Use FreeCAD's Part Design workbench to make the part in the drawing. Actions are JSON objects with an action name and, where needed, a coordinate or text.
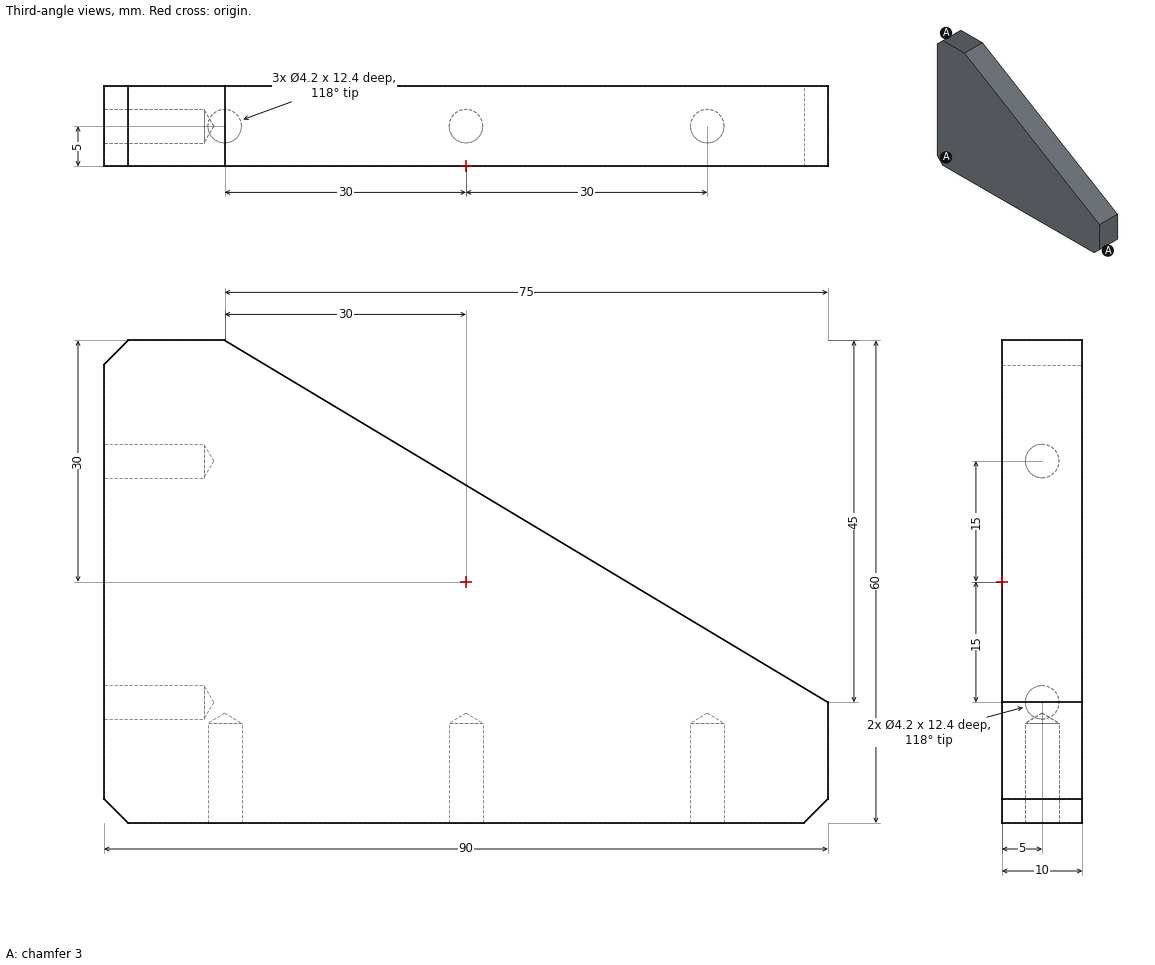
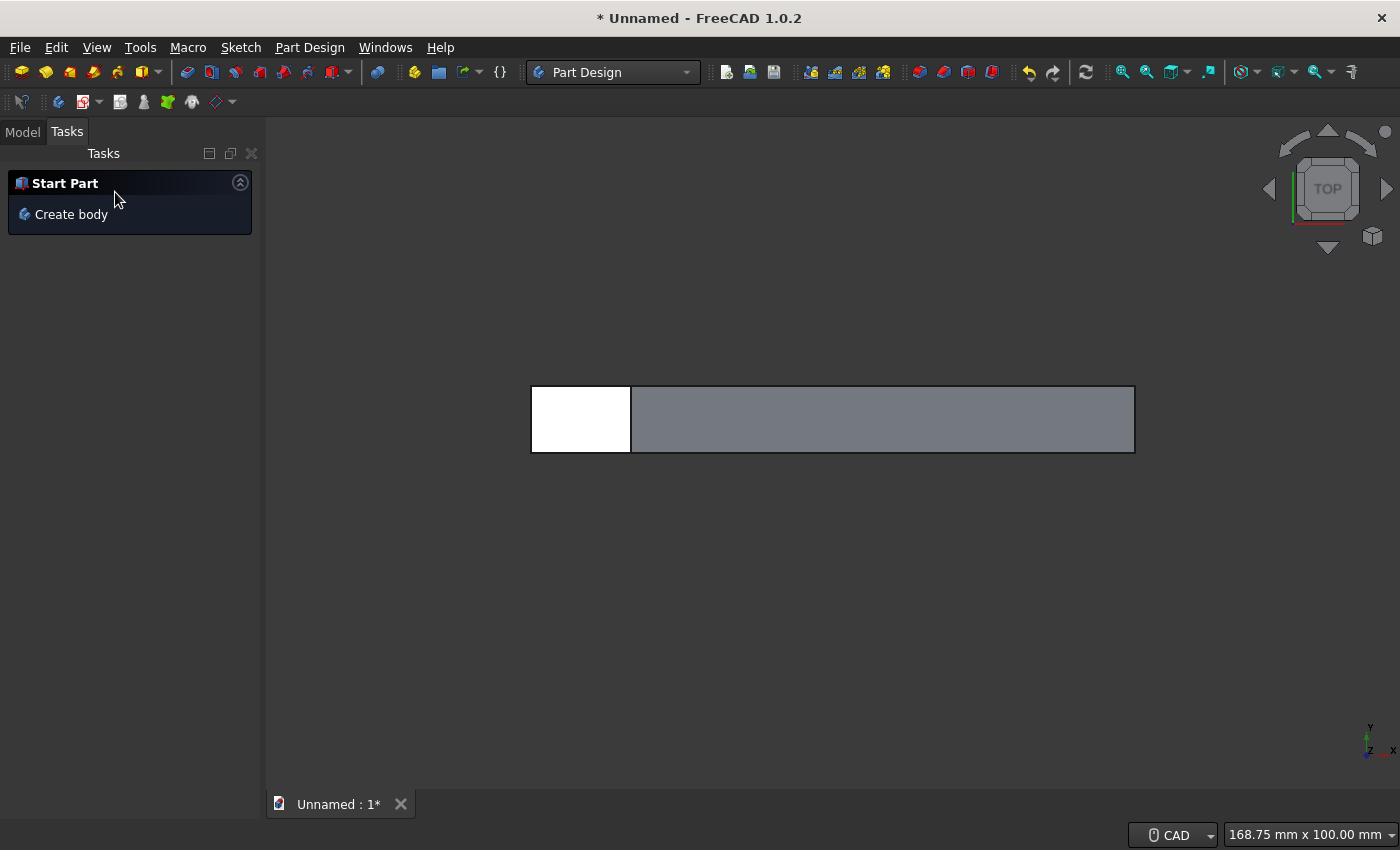
{"action": "left_click", "coordinate": [531, 418]}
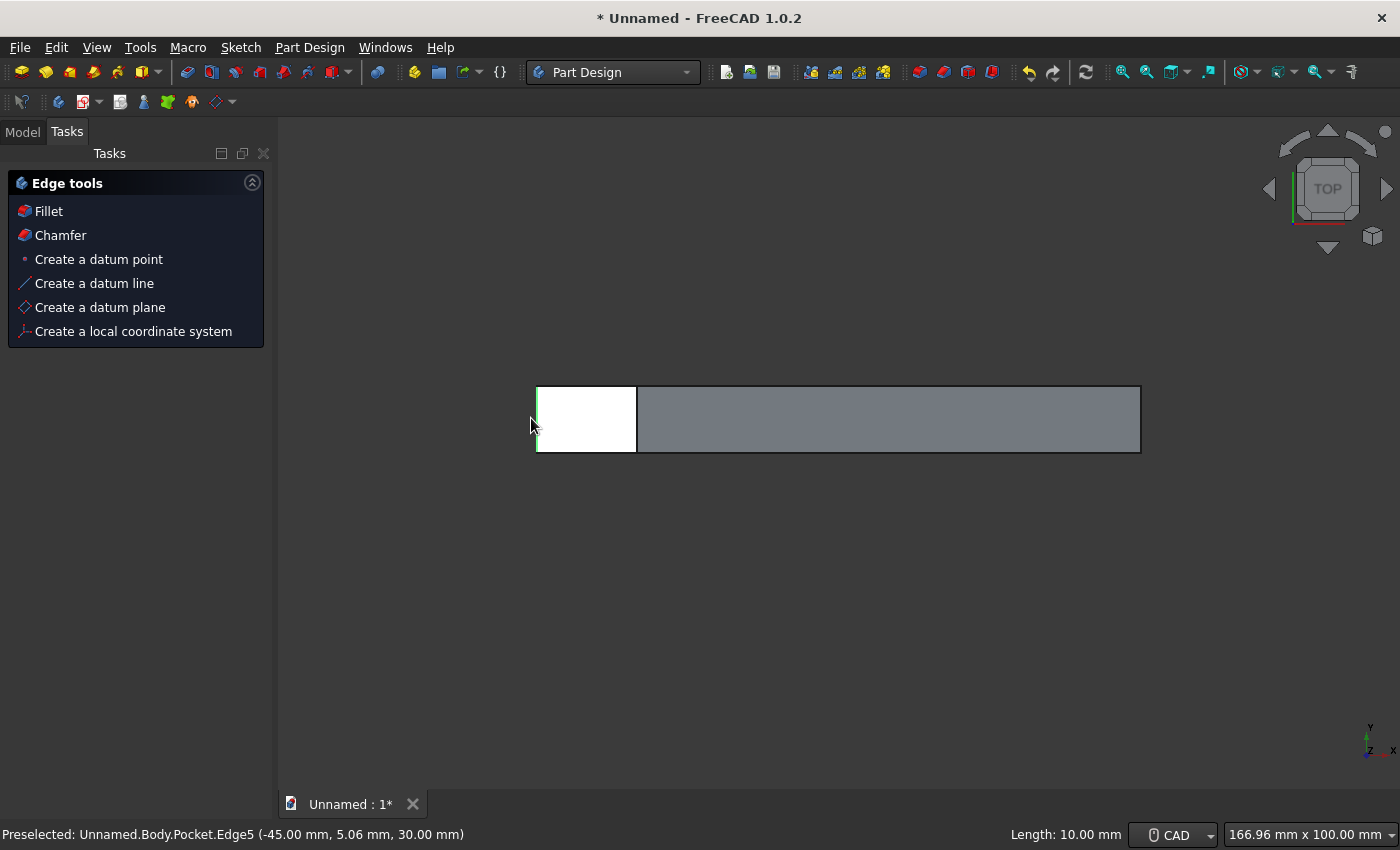
{"action": "key", "text": "1"}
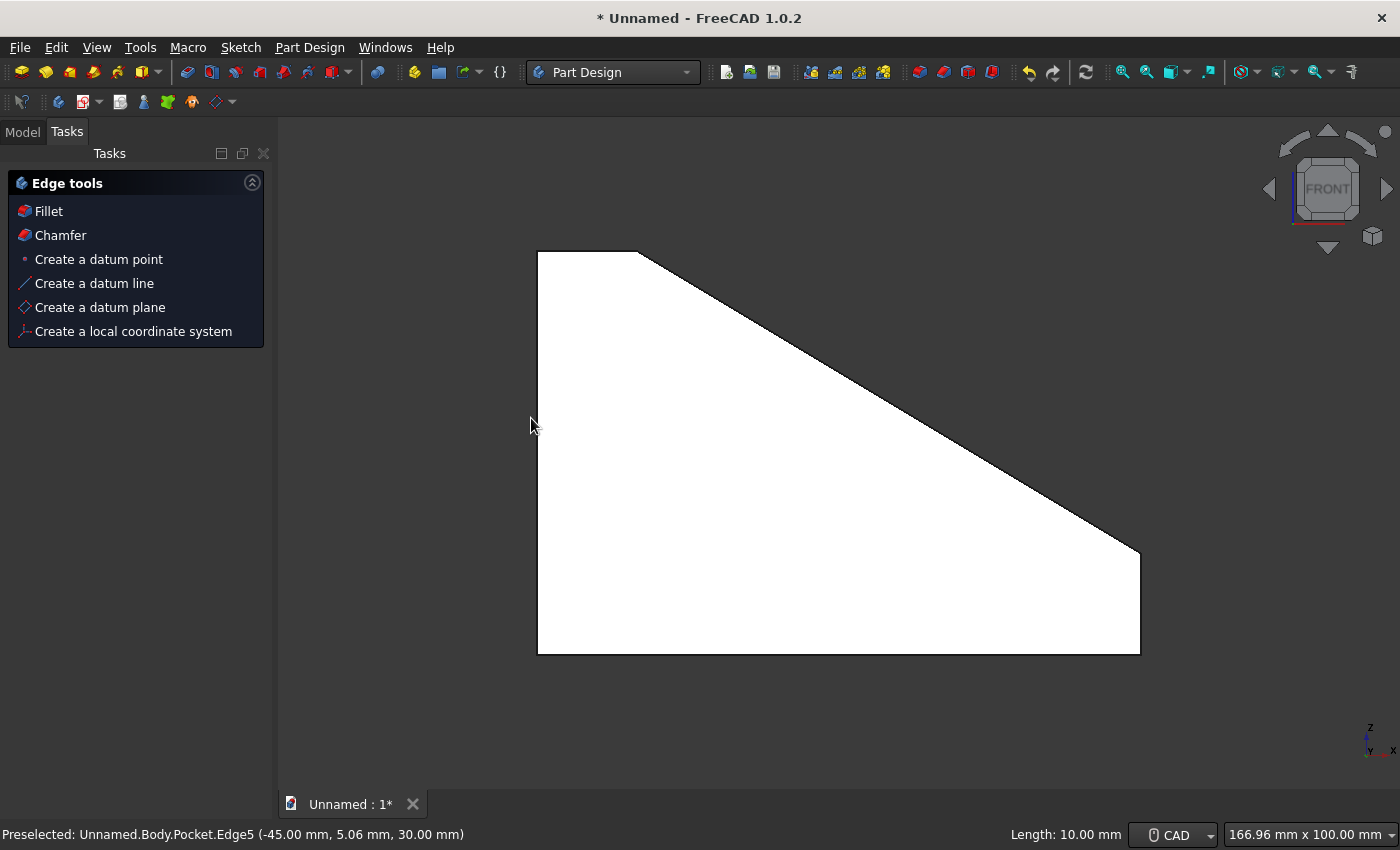
{"action": "key", "text": "3"}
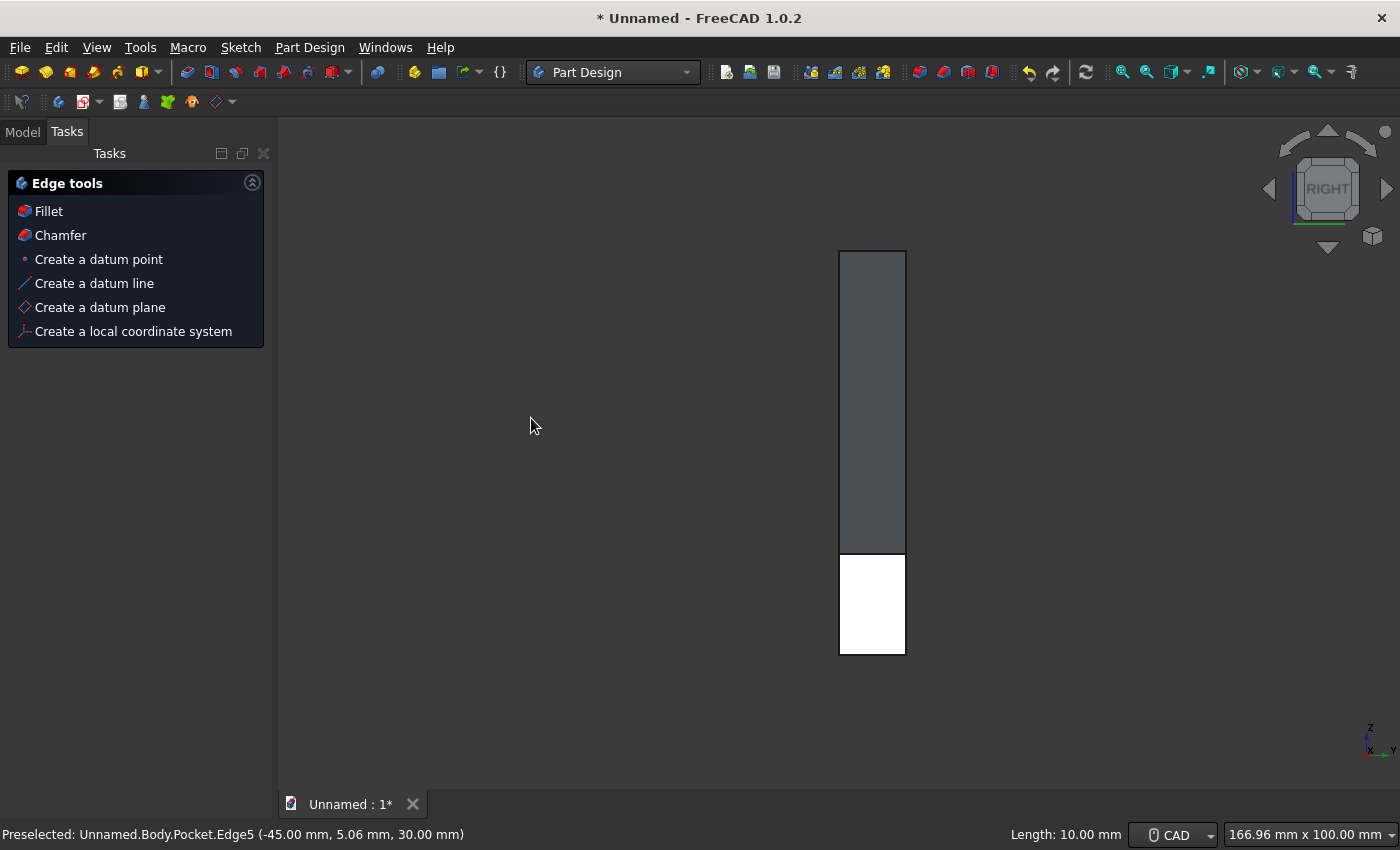
{"action": "left_click", "coordinate": [873, 654], "text": "ctrl"}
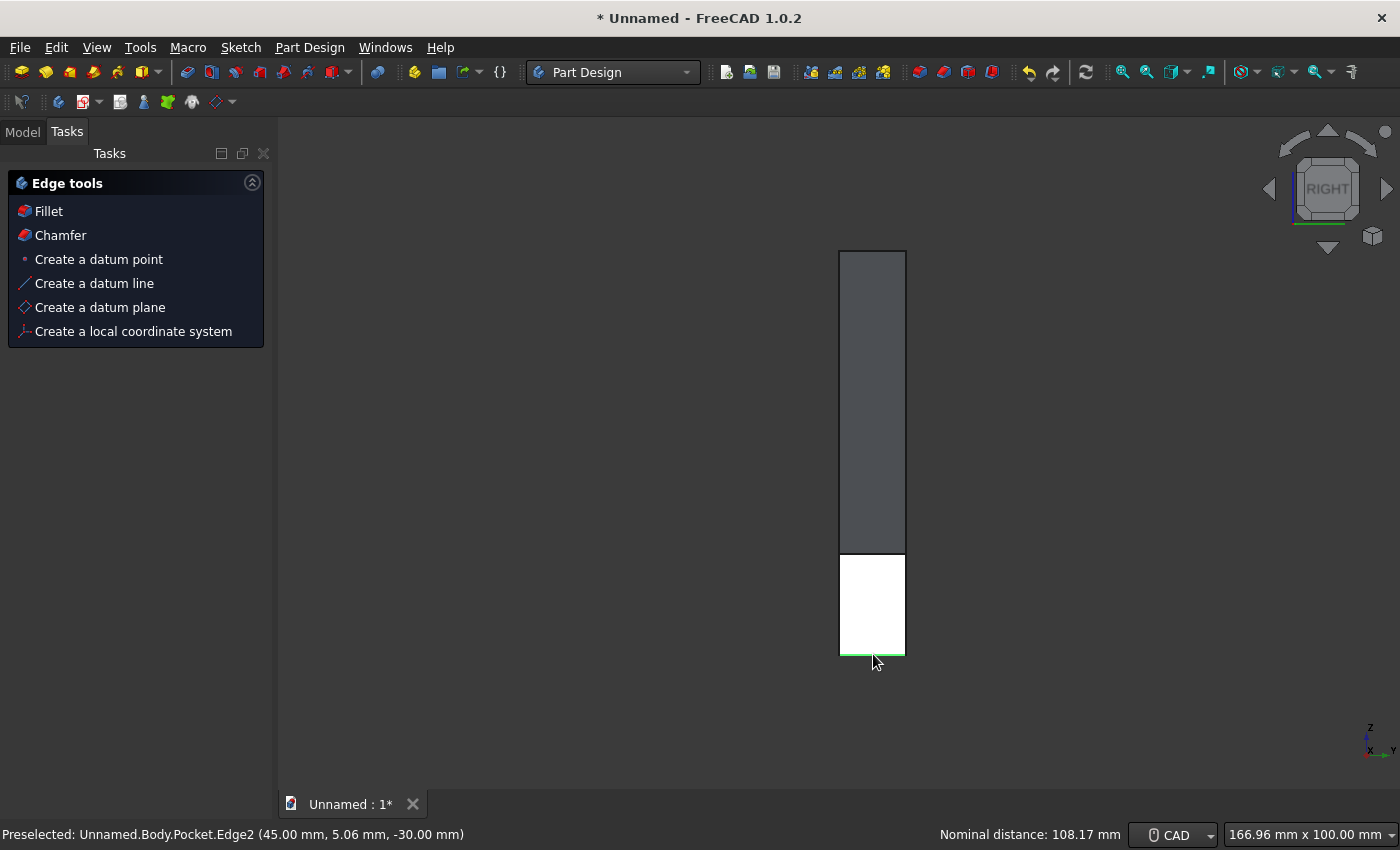
{"action": "key", "text": "5"}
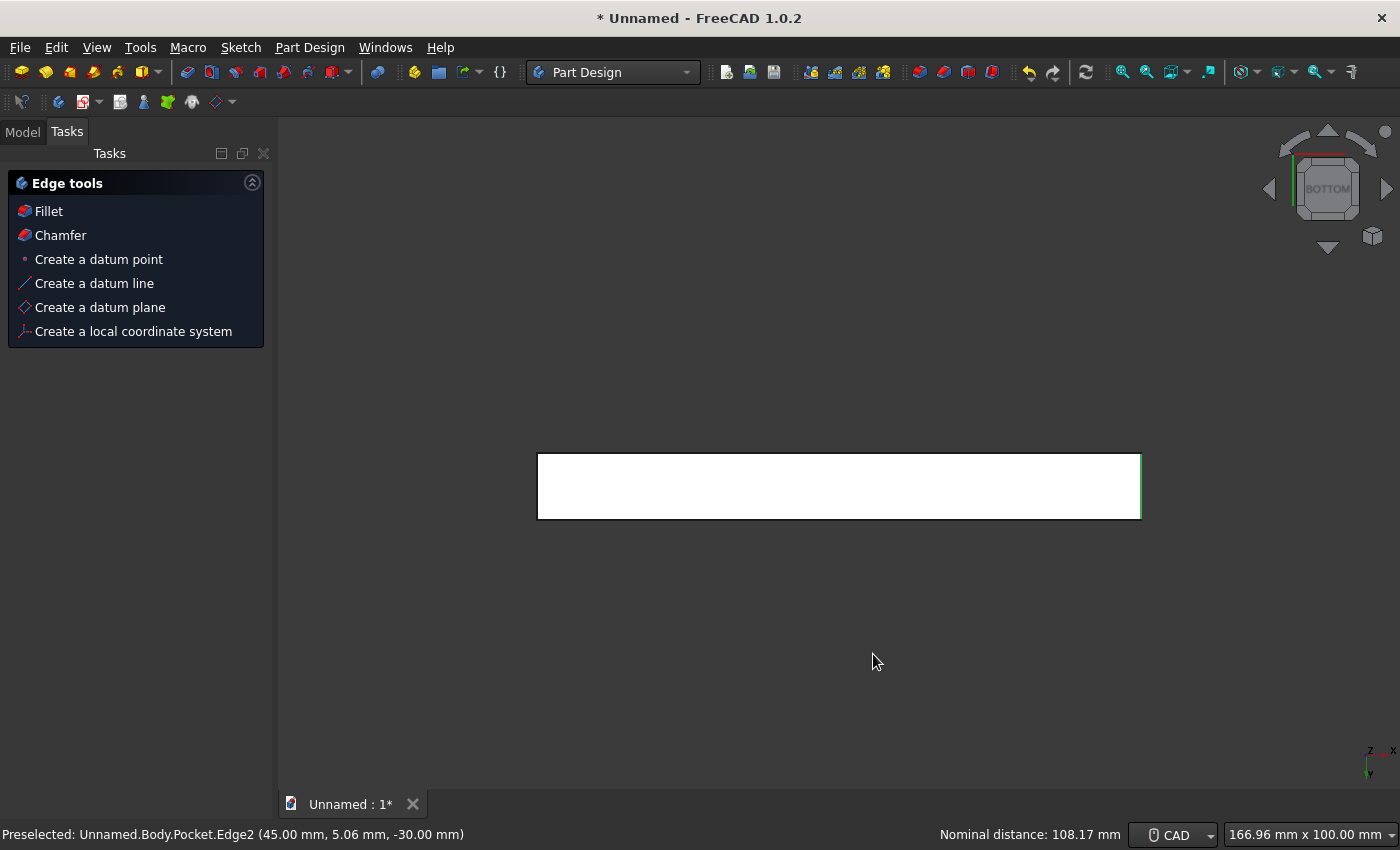
{"action": "left_click", "coordinate": [537, 486], "text": "ctrl"}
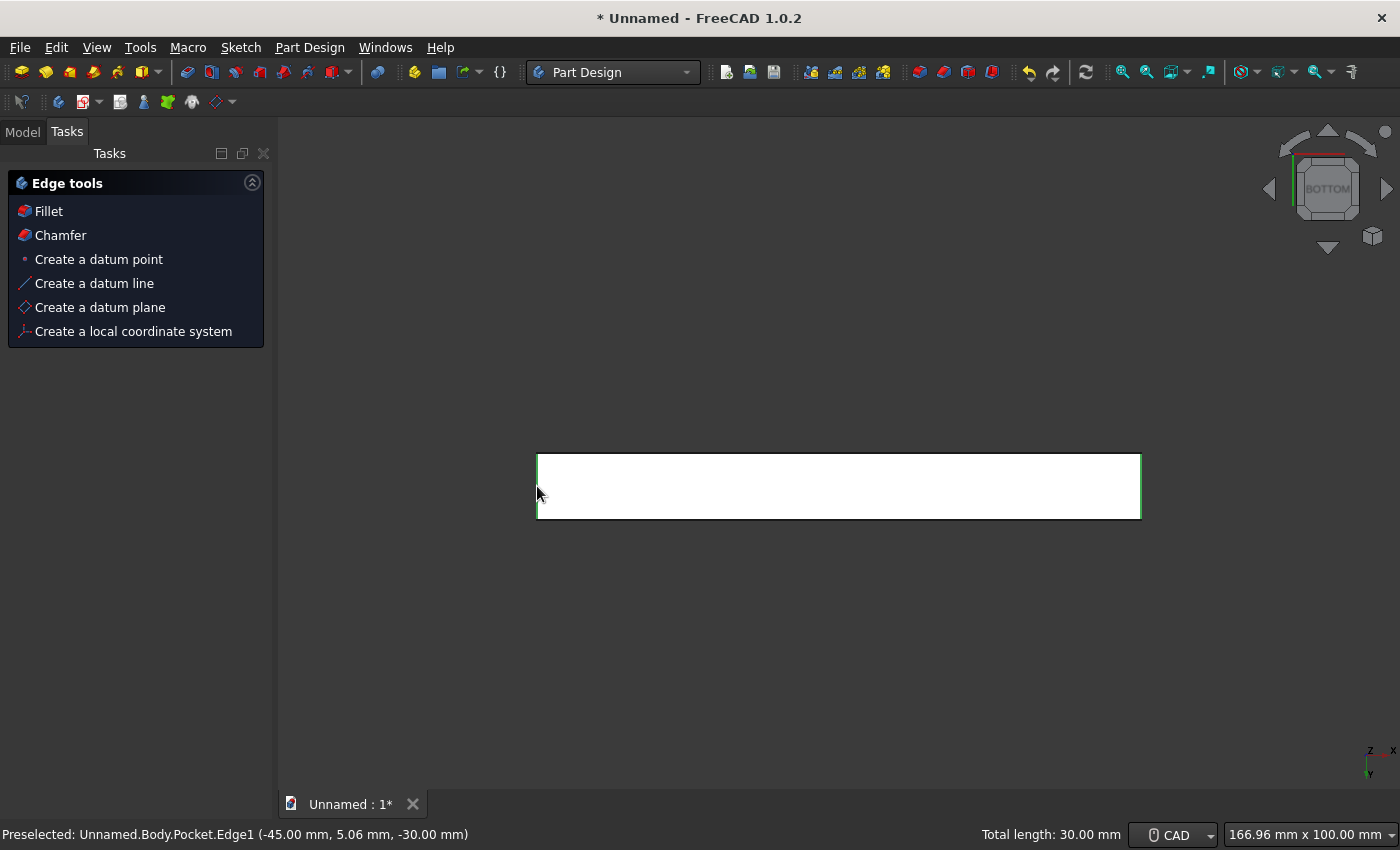
{"action": "left_click", "coordinate": [944, 72]}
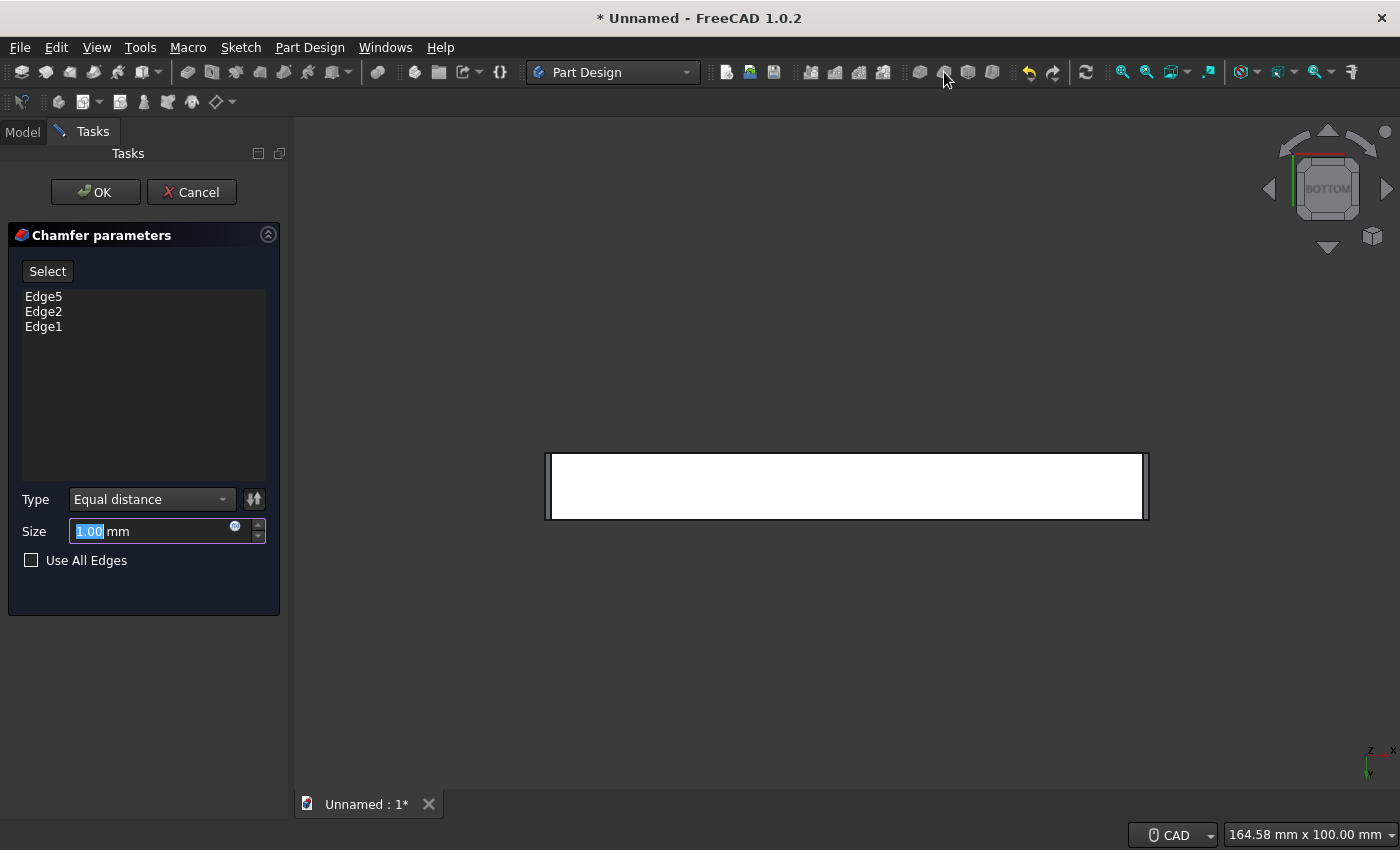
{"action": "type", "text": "3"}
{"action": "key", "text": "Tab"}